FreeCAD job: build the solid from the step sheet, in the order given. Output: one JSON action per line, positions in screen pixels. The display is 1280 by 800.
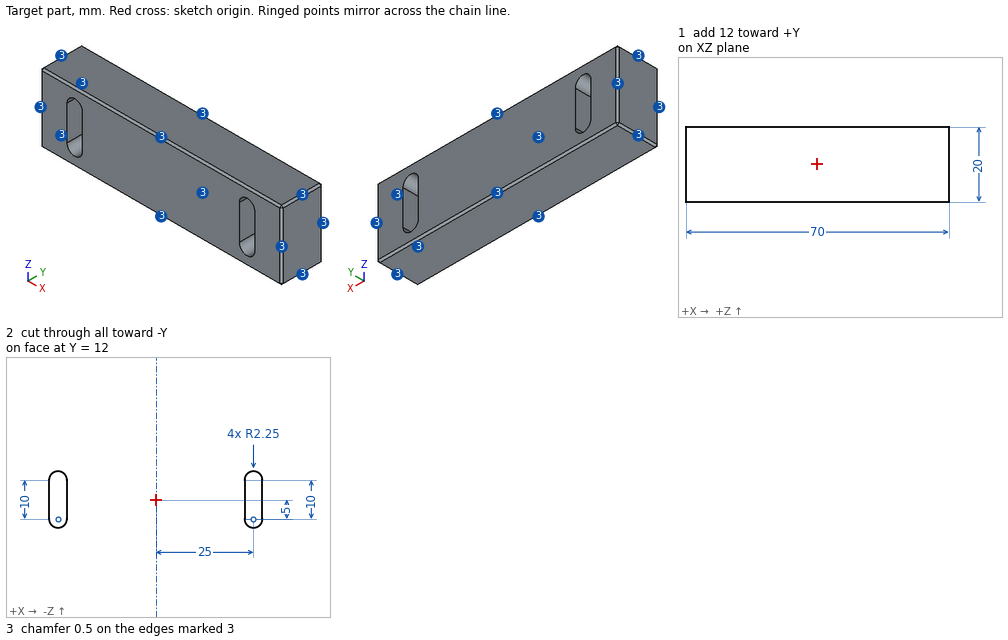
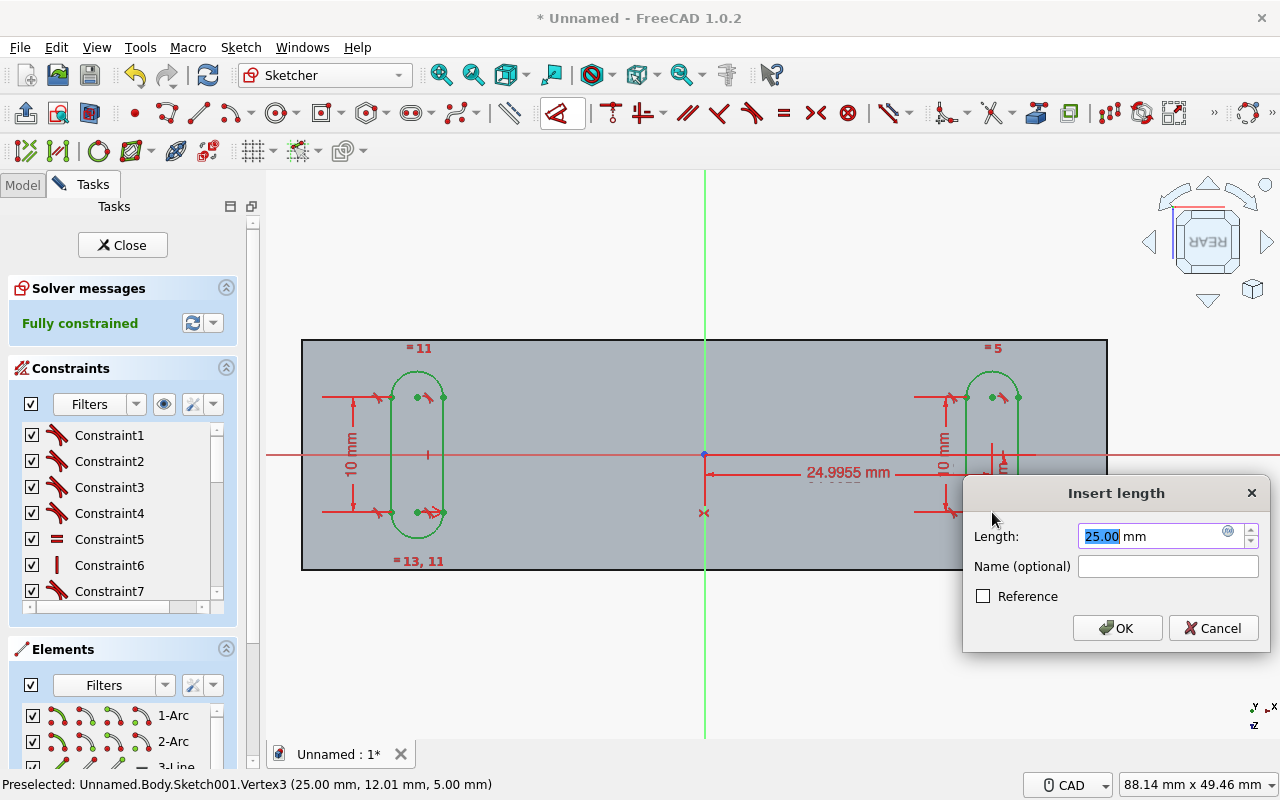
{"action": "type", "text": "25"}
{"action": "key", "text": "Return"}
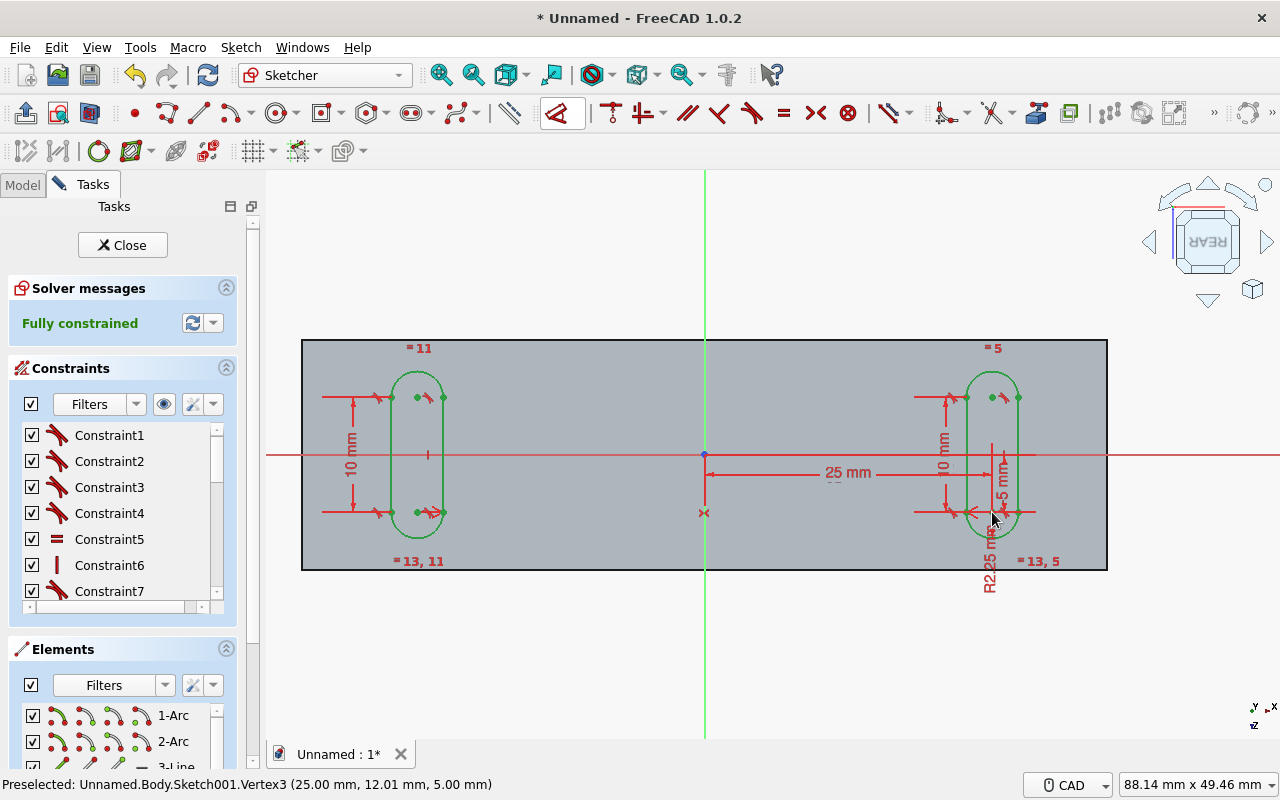
{"action": "left_click", "coordinate": [123, 245]}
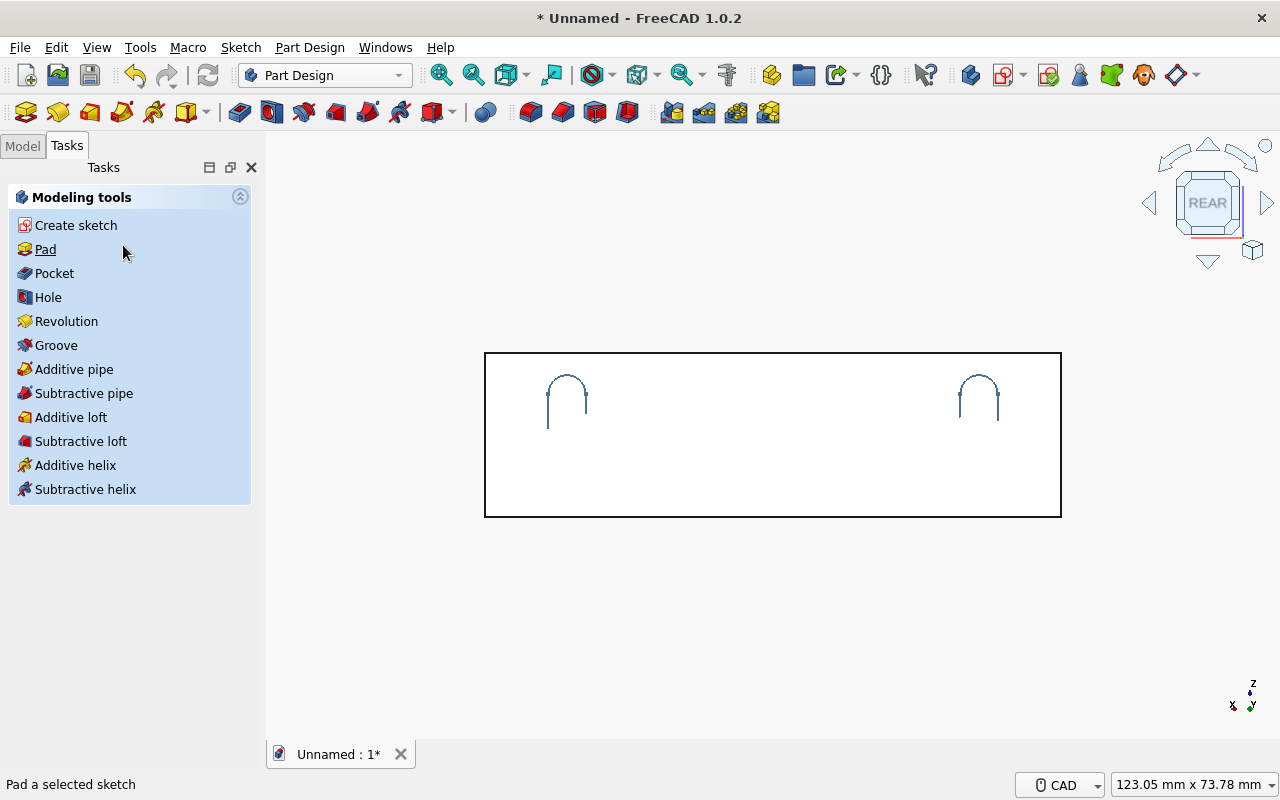
{"action": "left_click", "coordinate": [240, 112]}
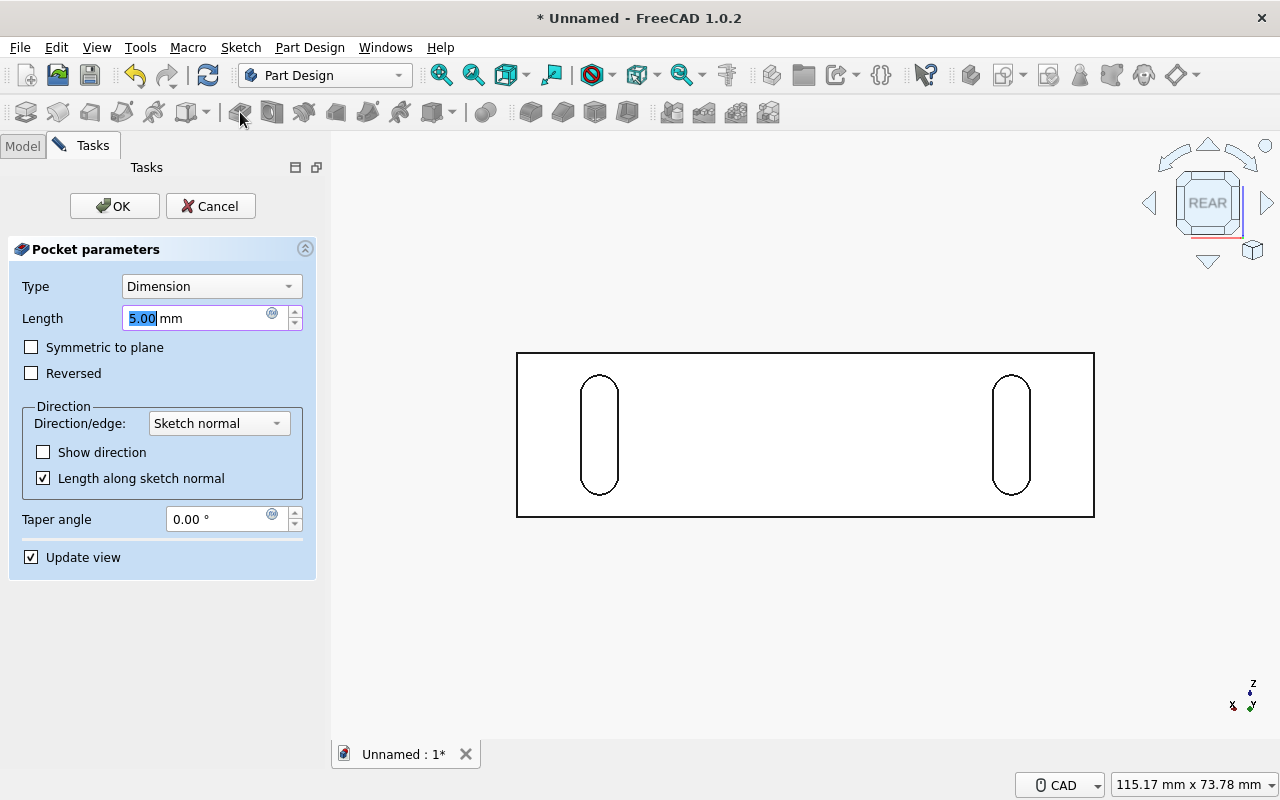
{"action": "left_click", "coordinate": [212, 286]}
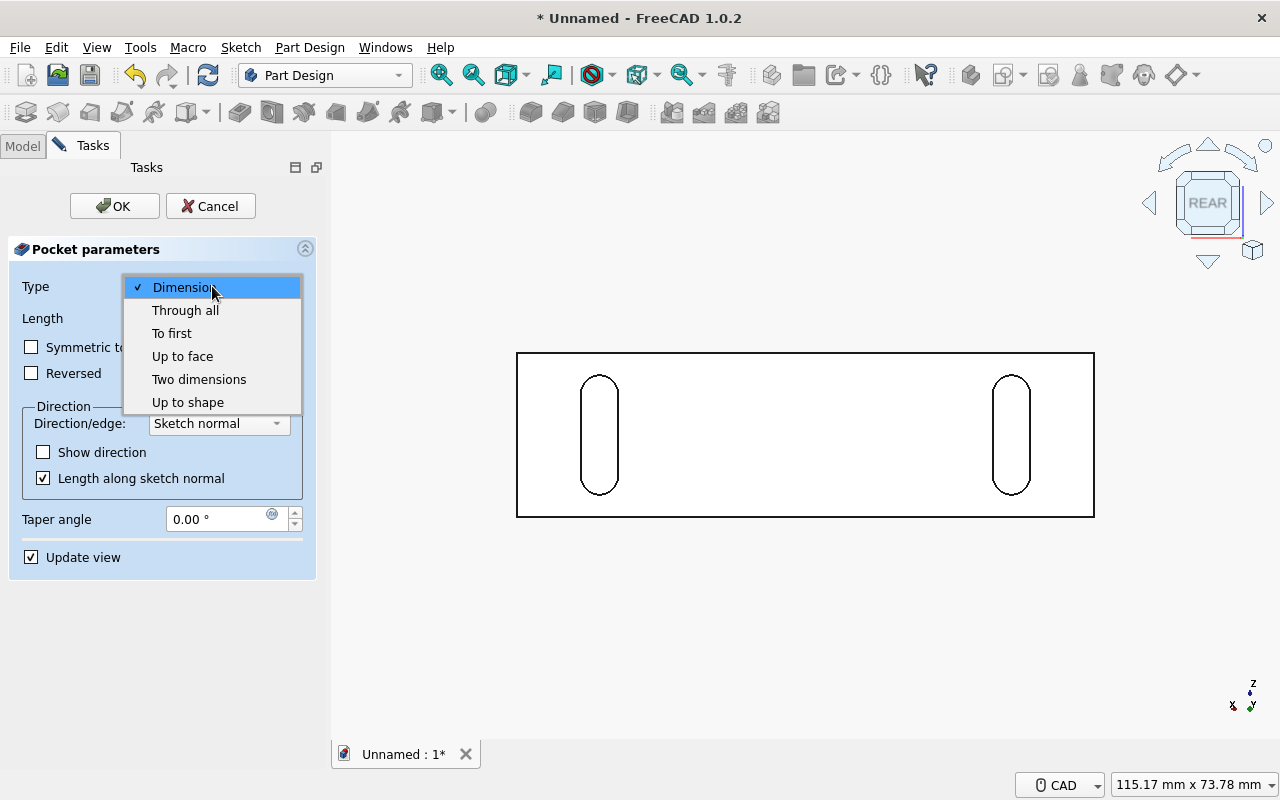
{"action": "left_click", "coordinate": [212, 310]}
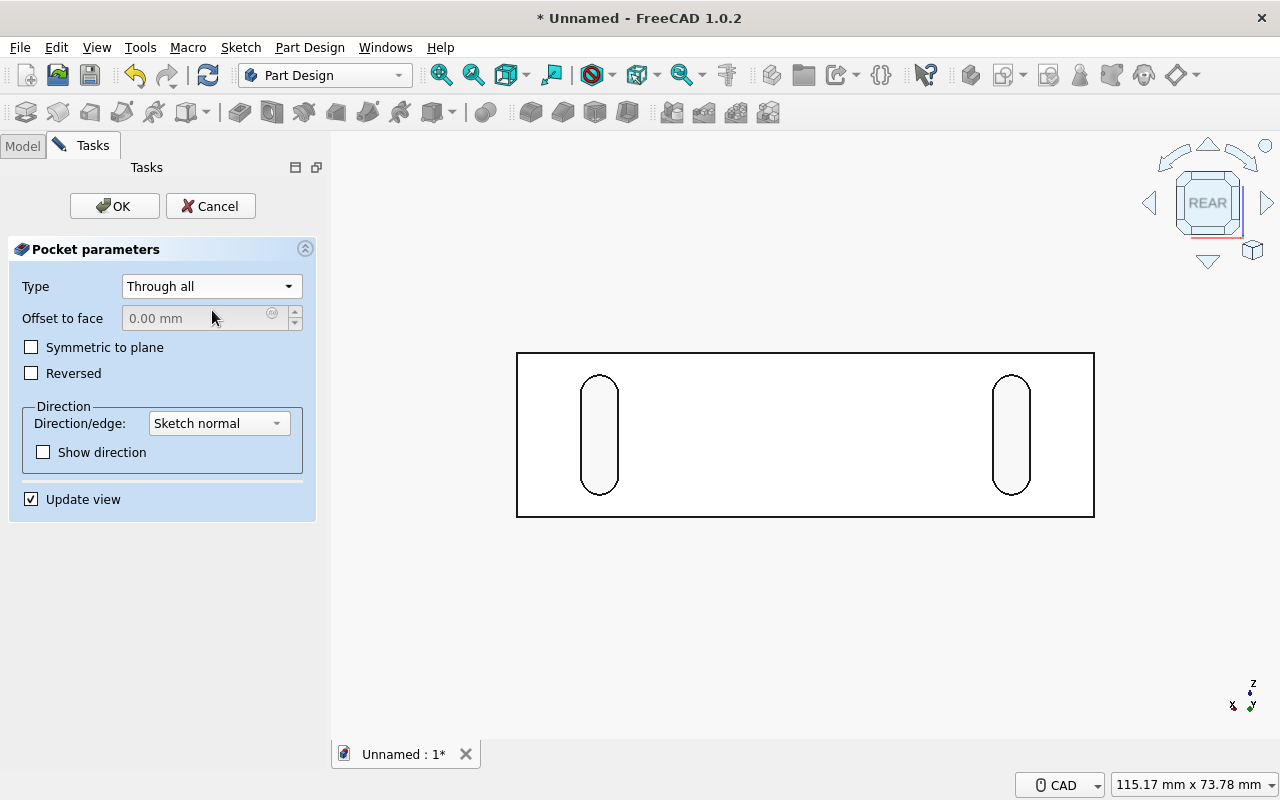
{"action": "left_click", "coordinate": [115, 206]}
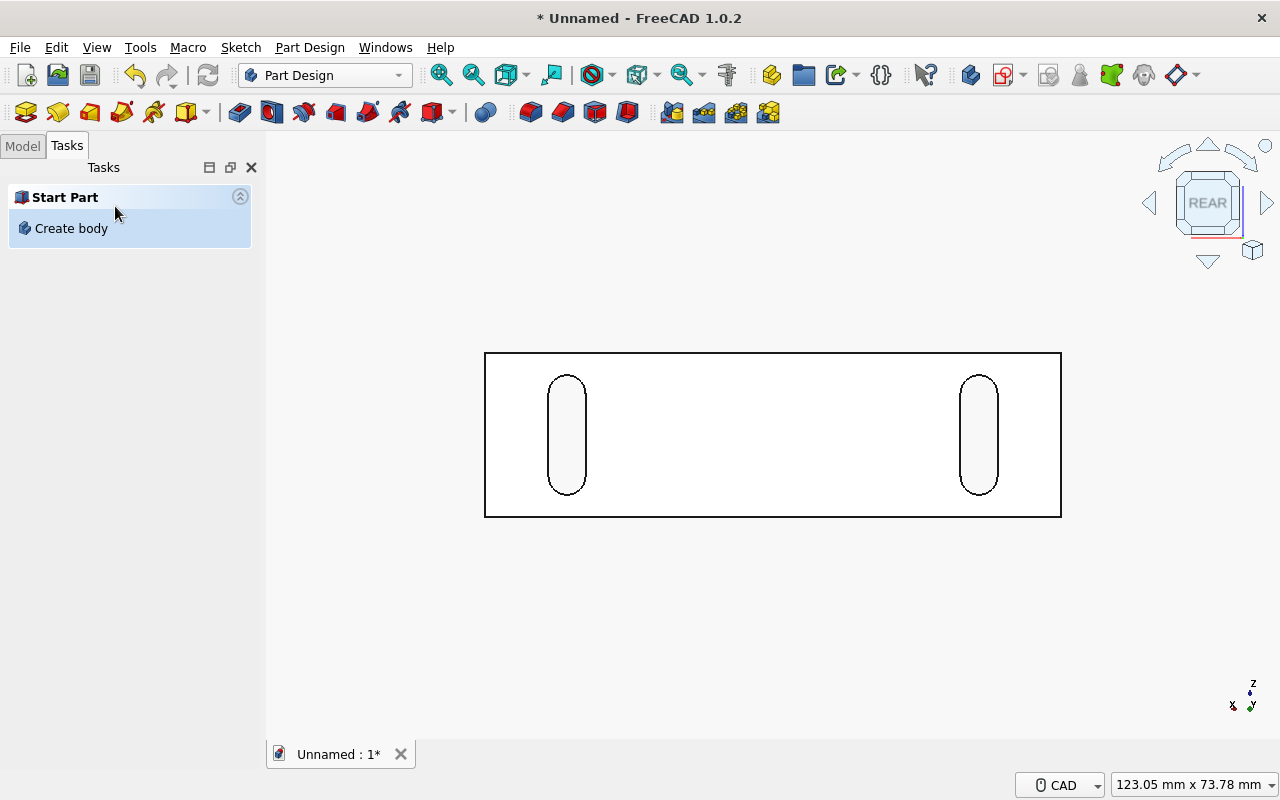
{"action": "left_click", "coordinate": [1061, 434]}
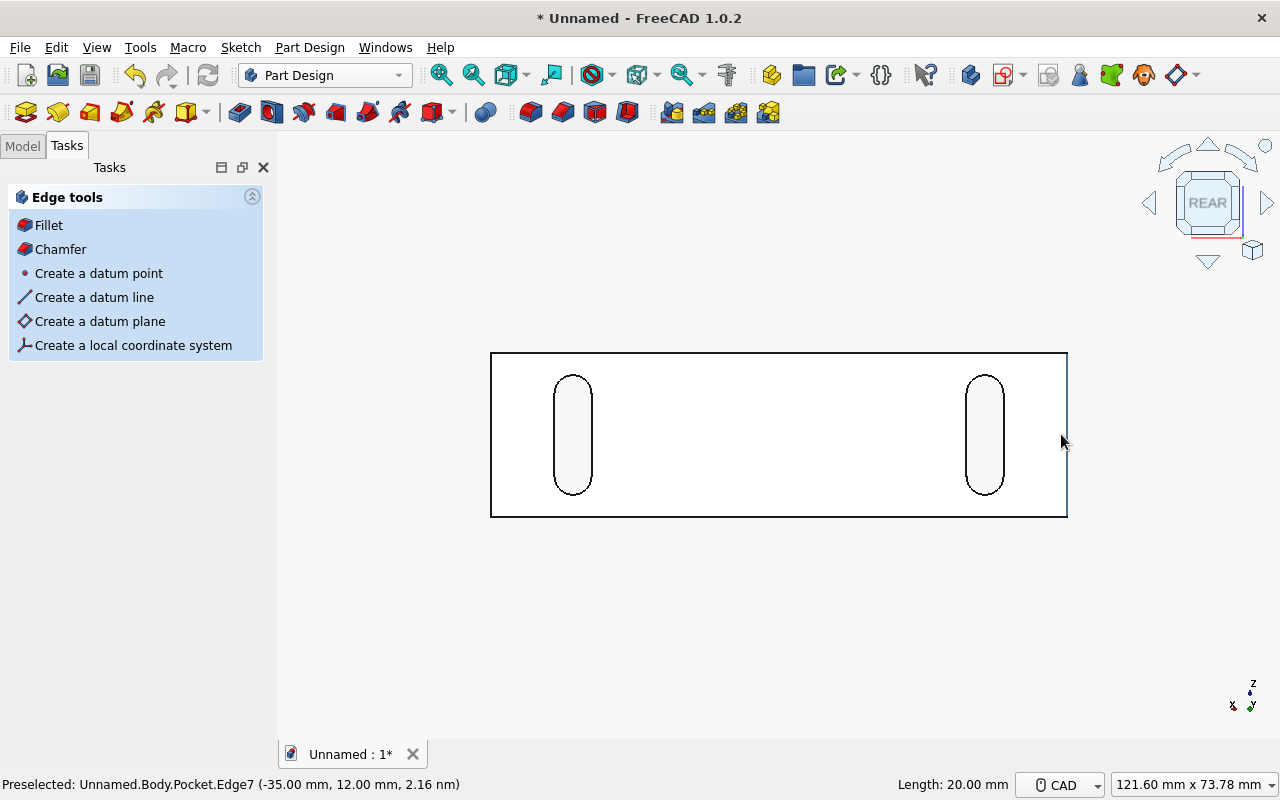
{"action": "key", "text": "0"}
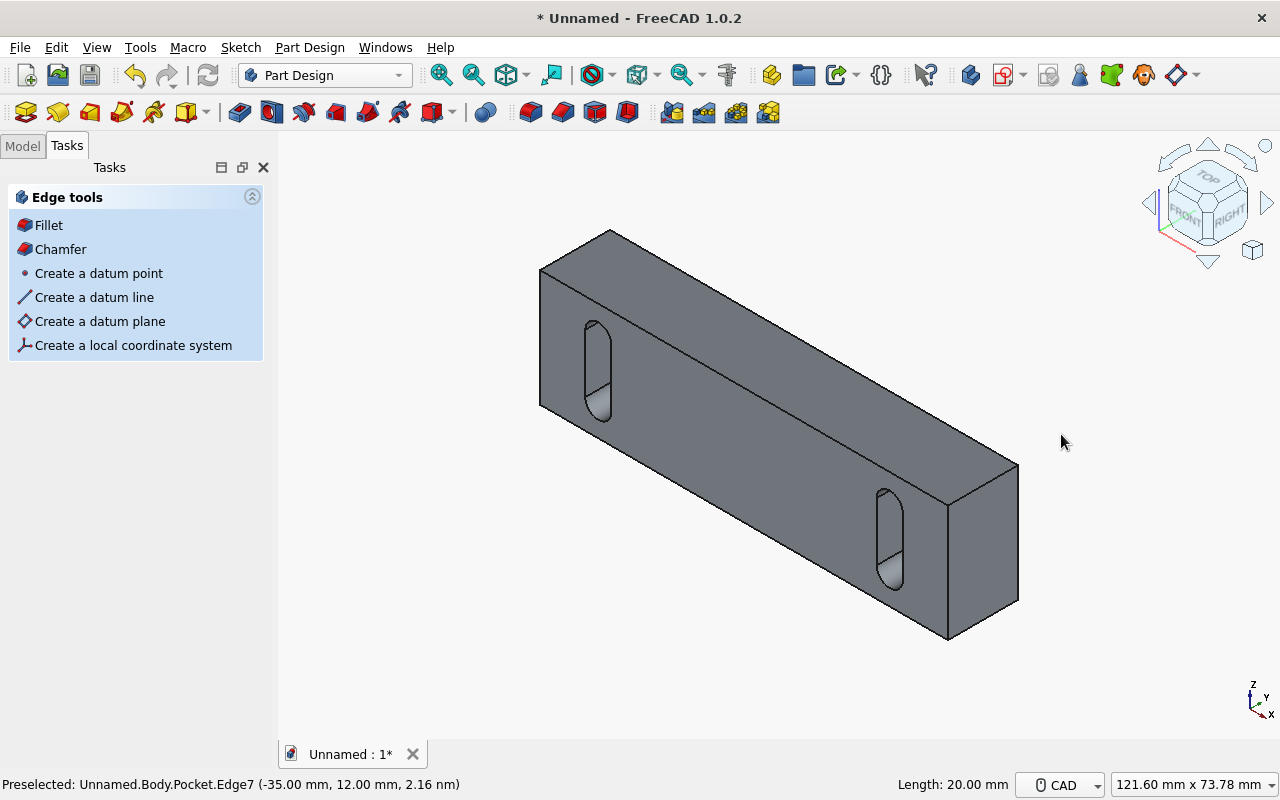
{"action": "left_click", "coordinate": [896, 434], "text": "ctrl"}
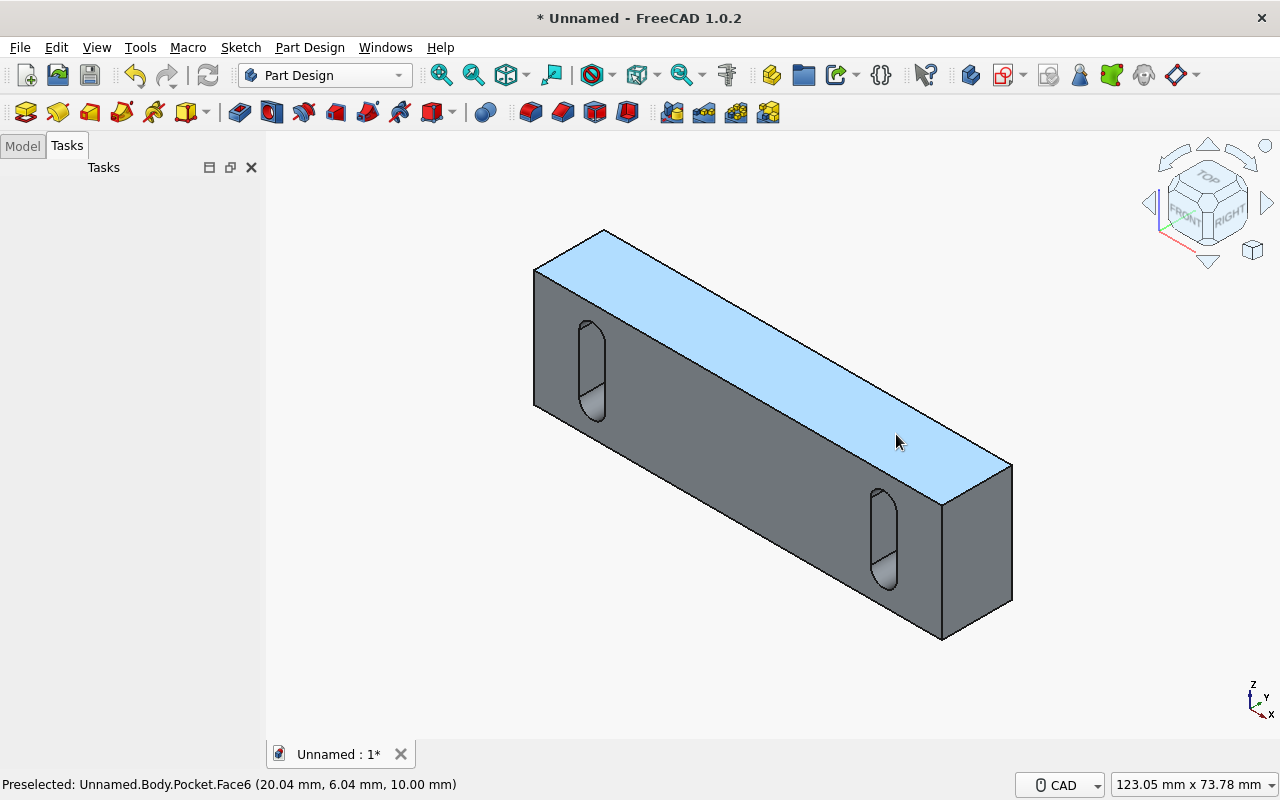
{"action": "left_click", "coordinate": [942, 572], "text": "ctrl"}